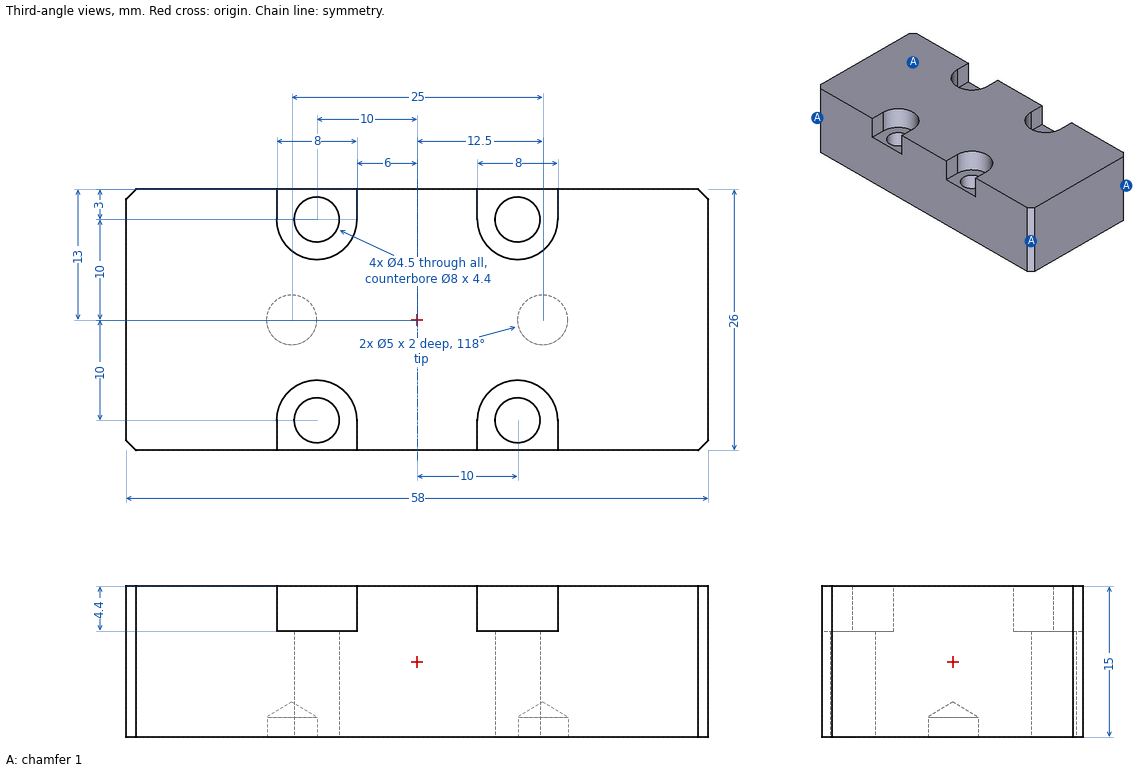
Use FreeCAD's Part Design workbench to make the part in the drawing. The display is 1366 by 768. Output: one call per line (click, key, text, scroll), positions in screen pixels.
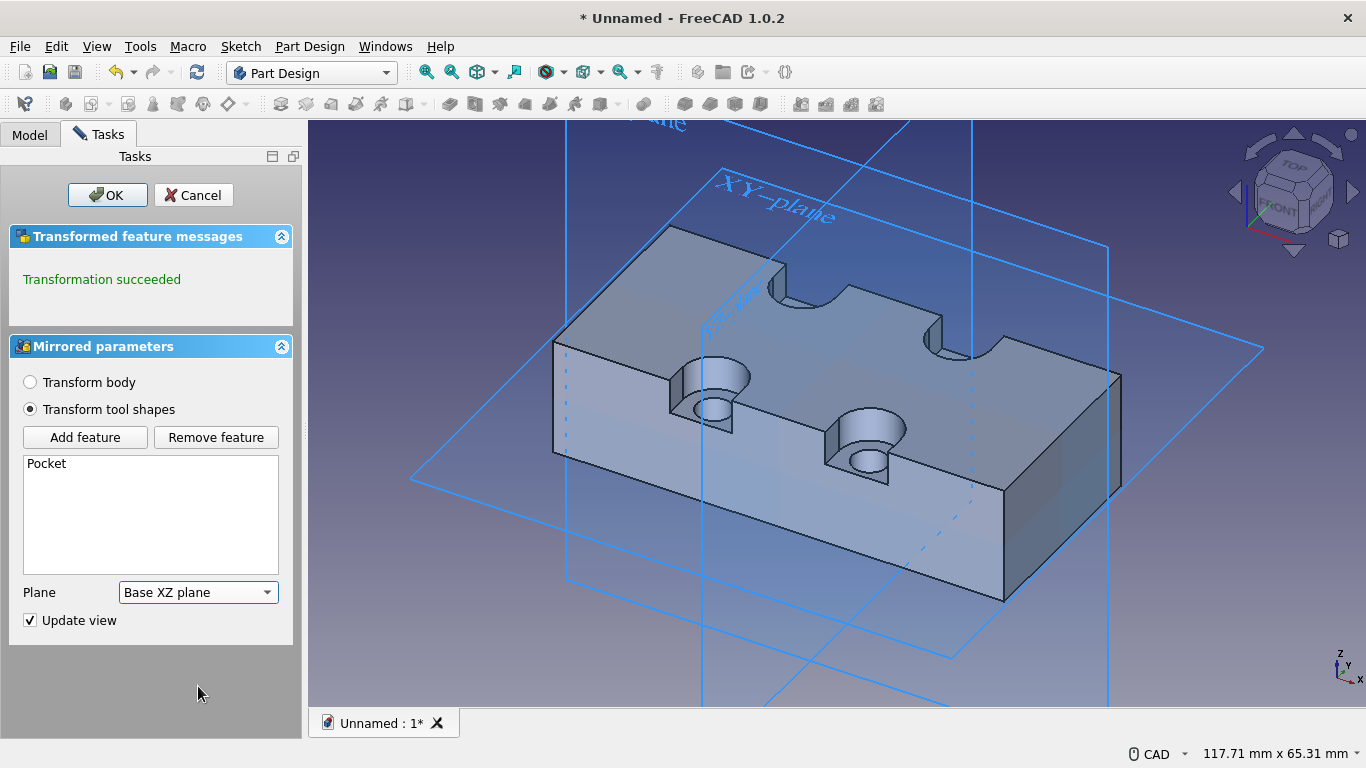
click(108, 195)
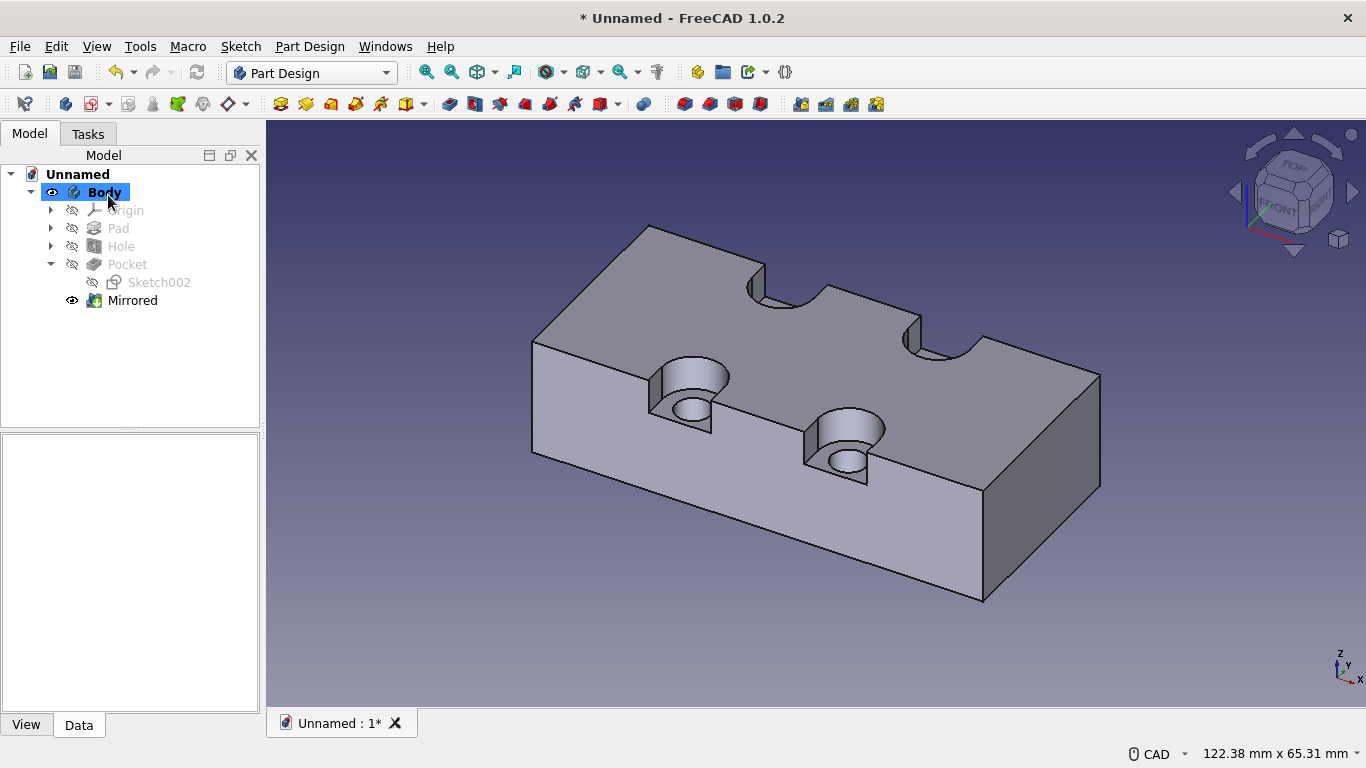
key(5)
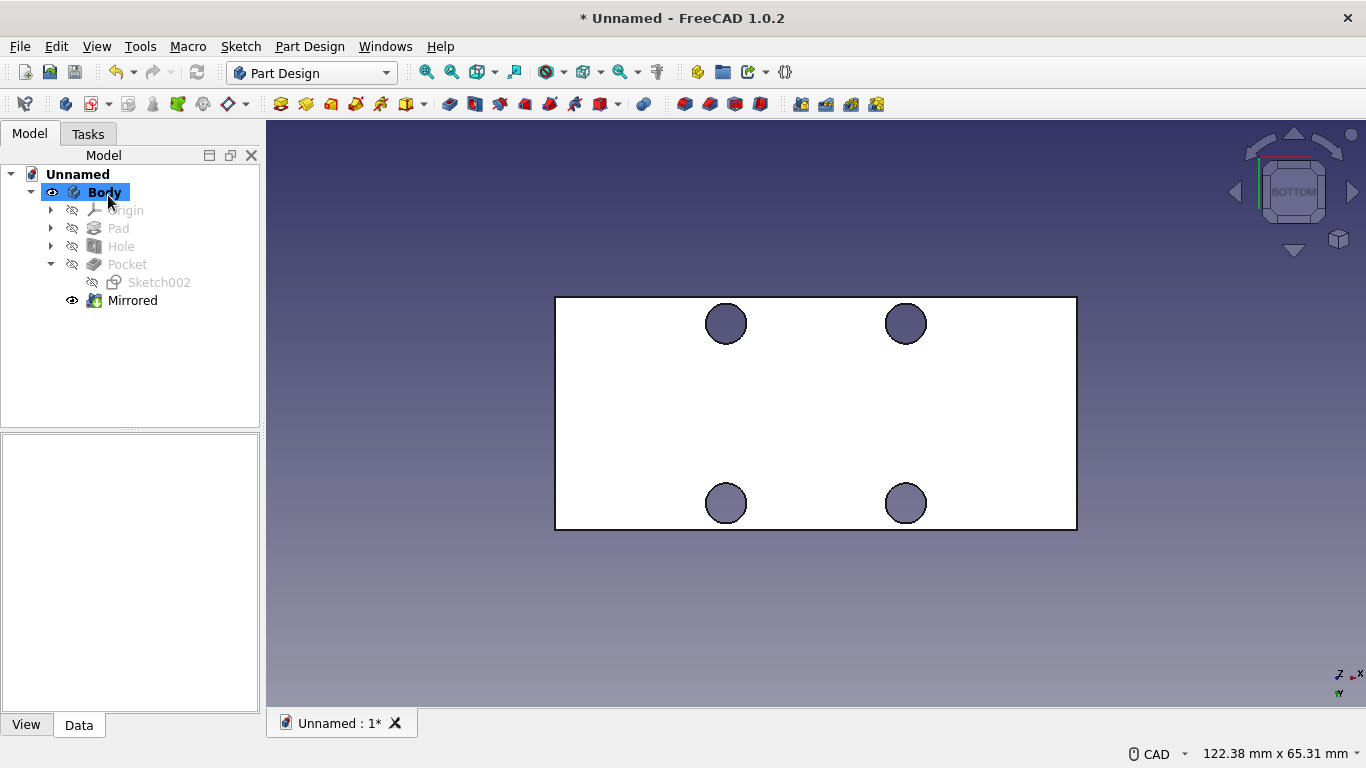
click(816, 413)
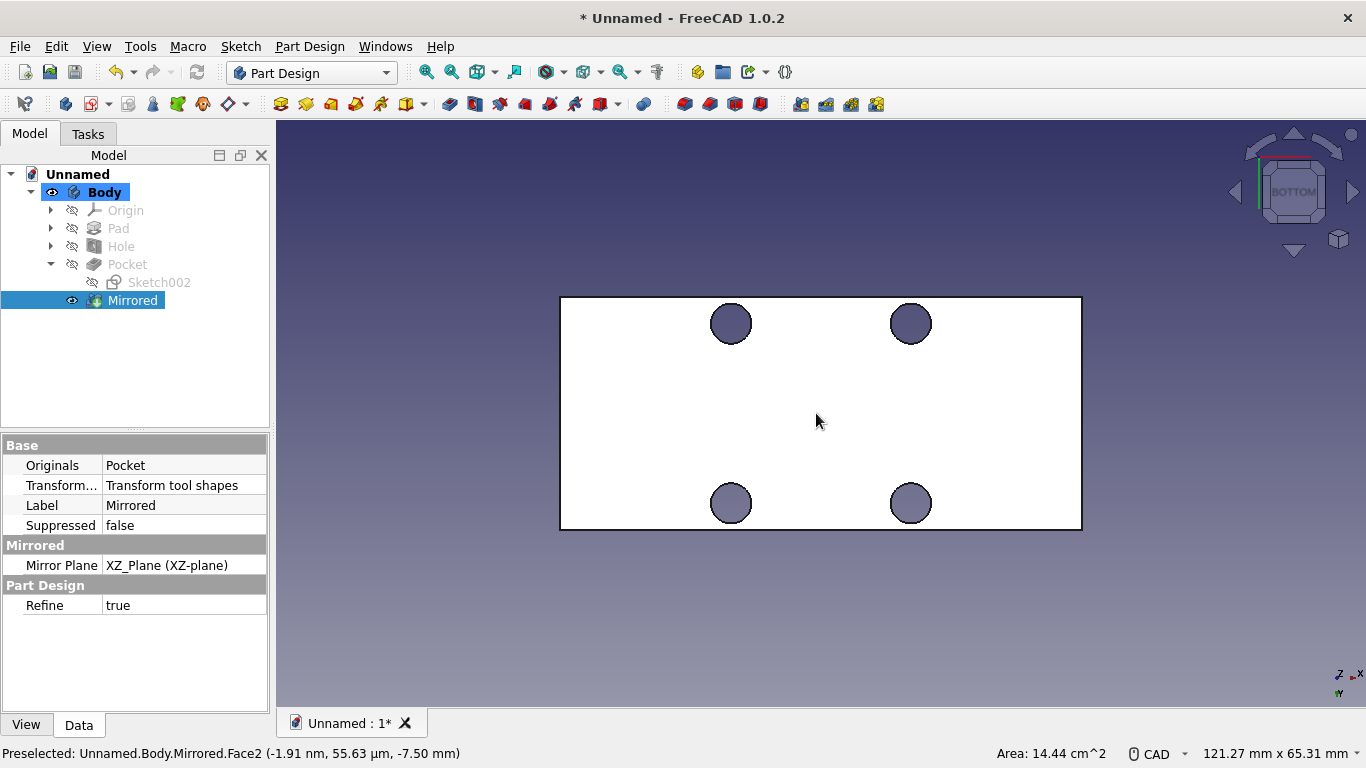
click(90, 104)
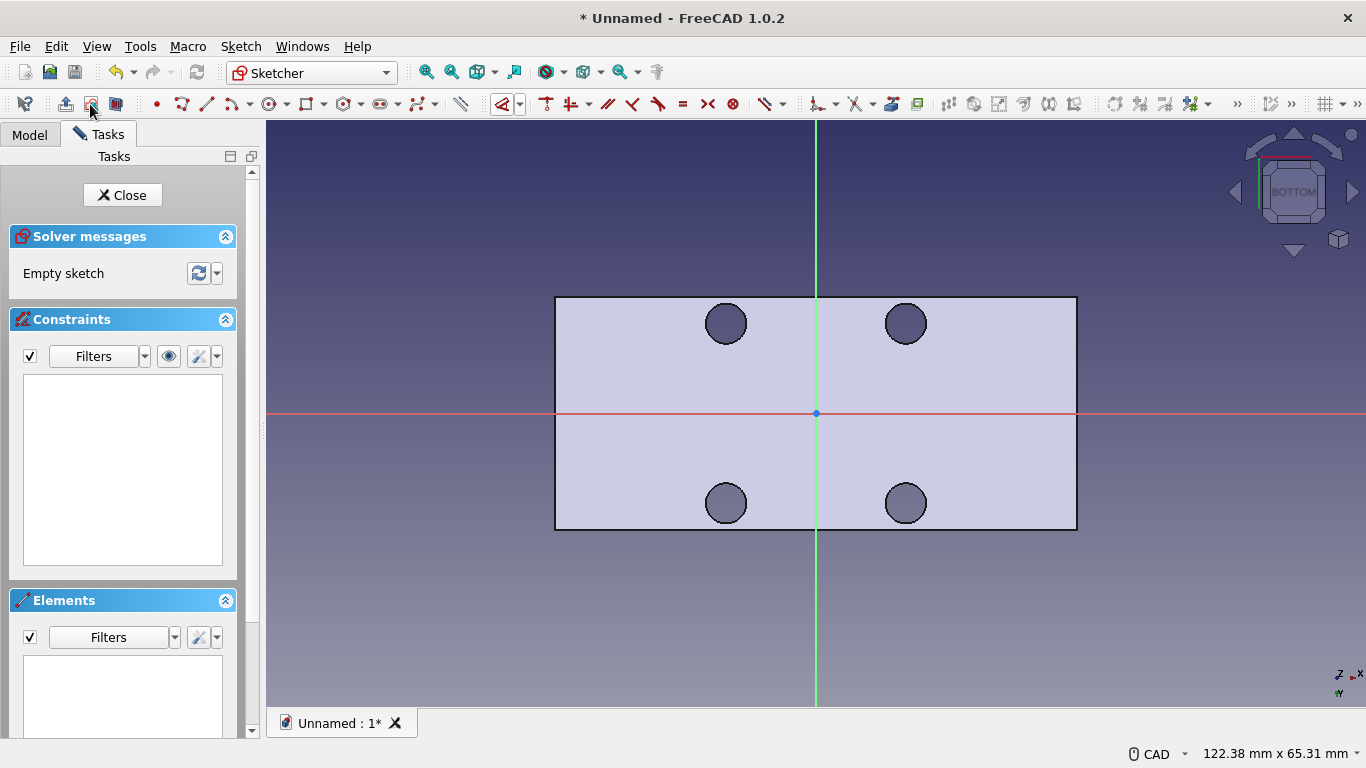
scroll(872, 414, up, 4)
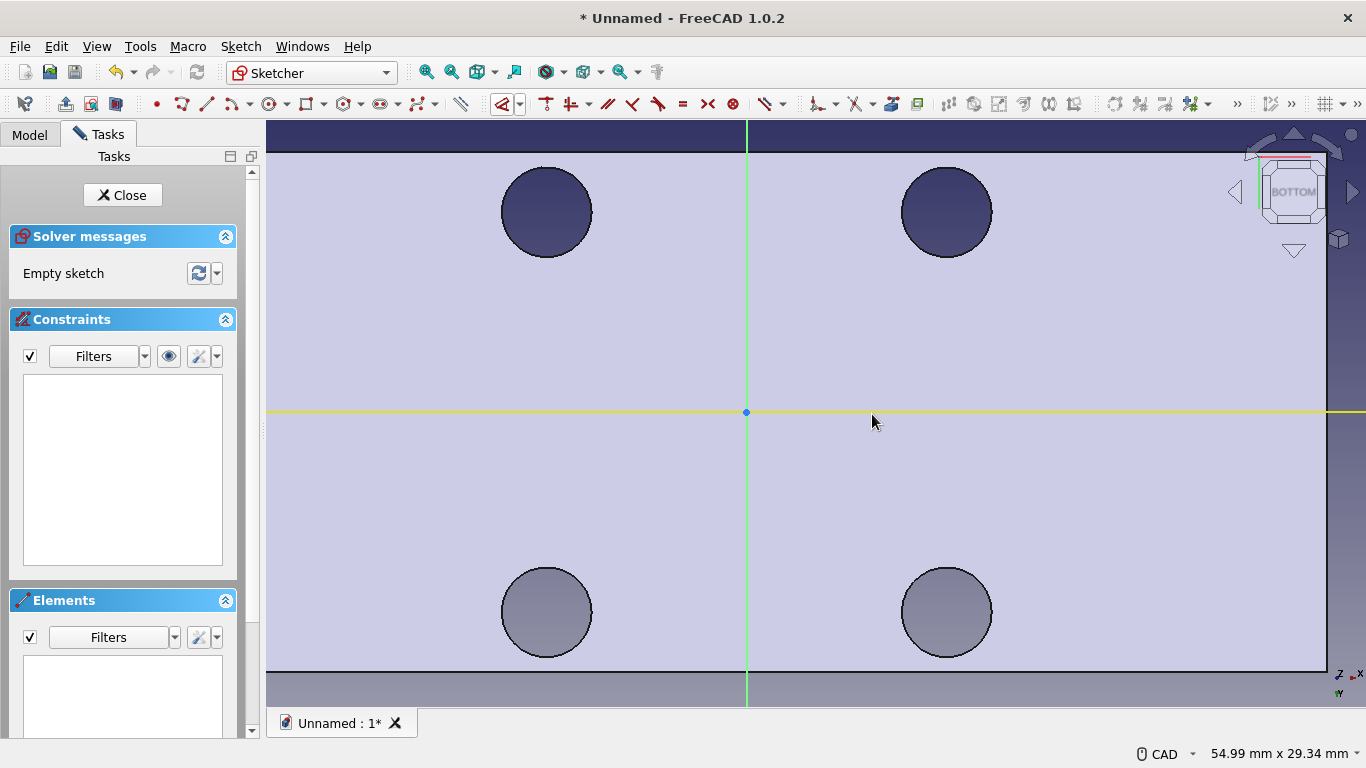
click(268, 104)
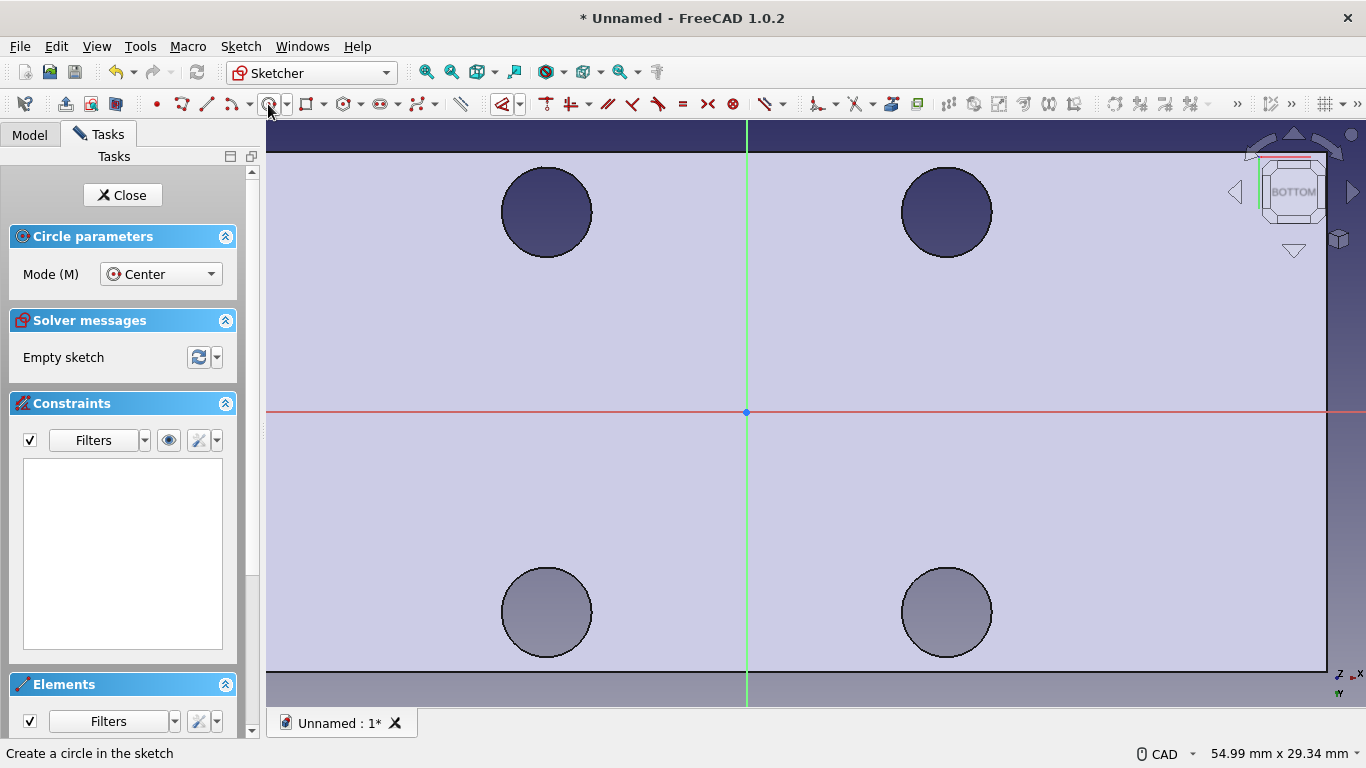
click(997, 412)
move(1032, 377)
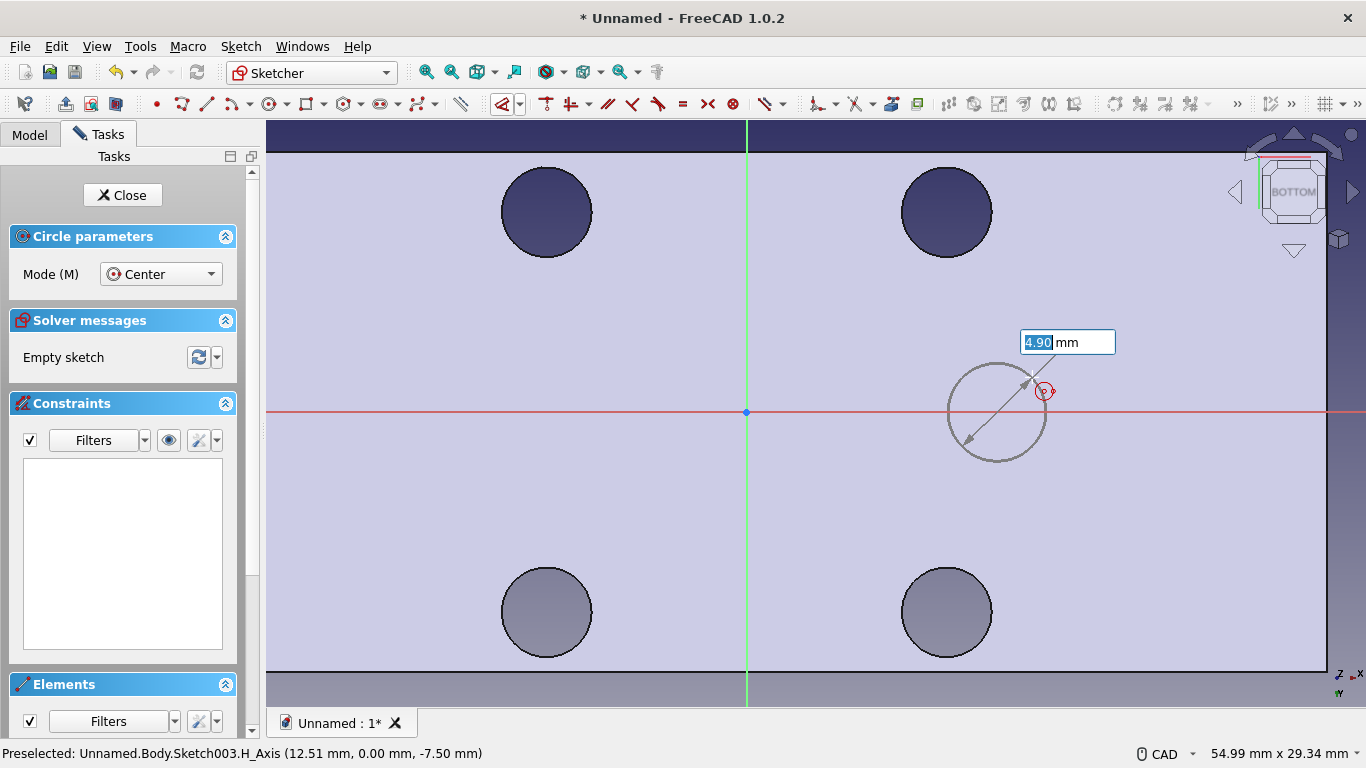
text(5)
key(Return)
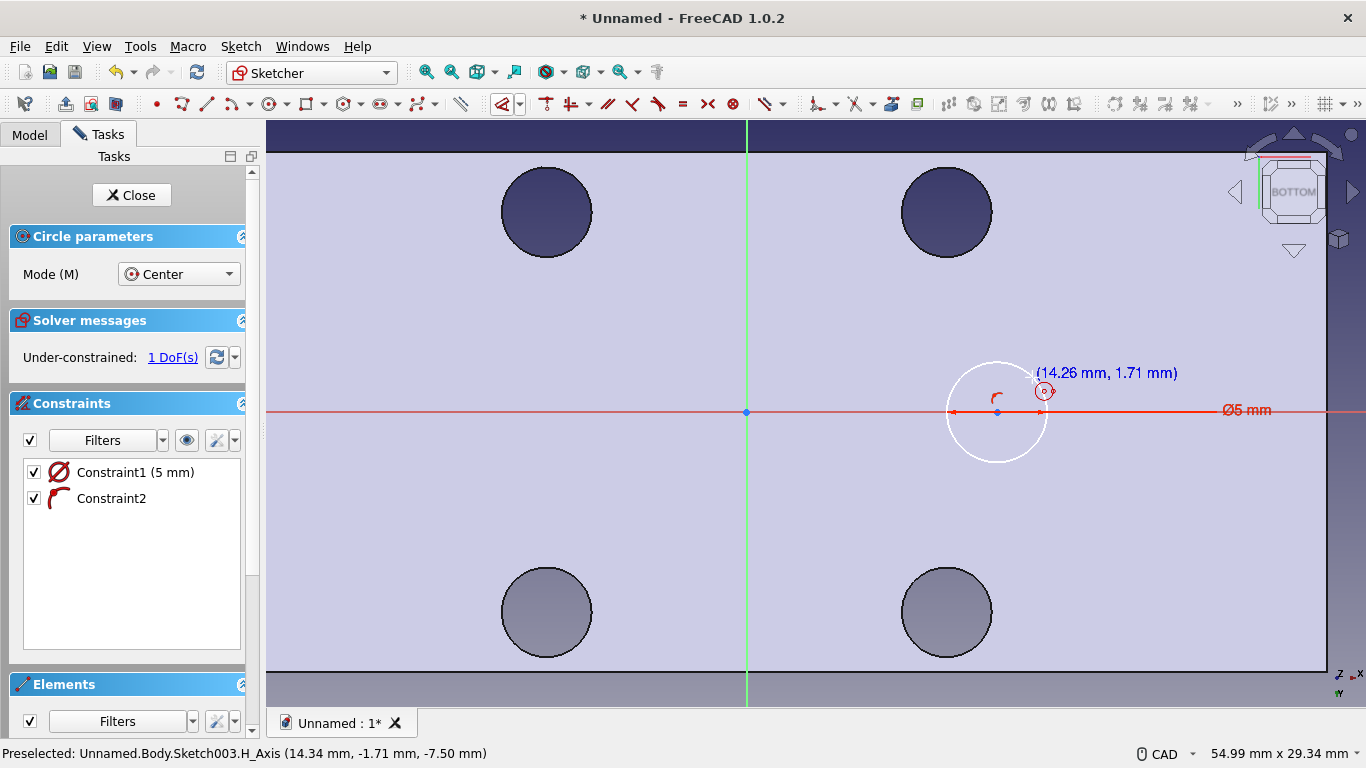
click(497, 412)
move(532, 377)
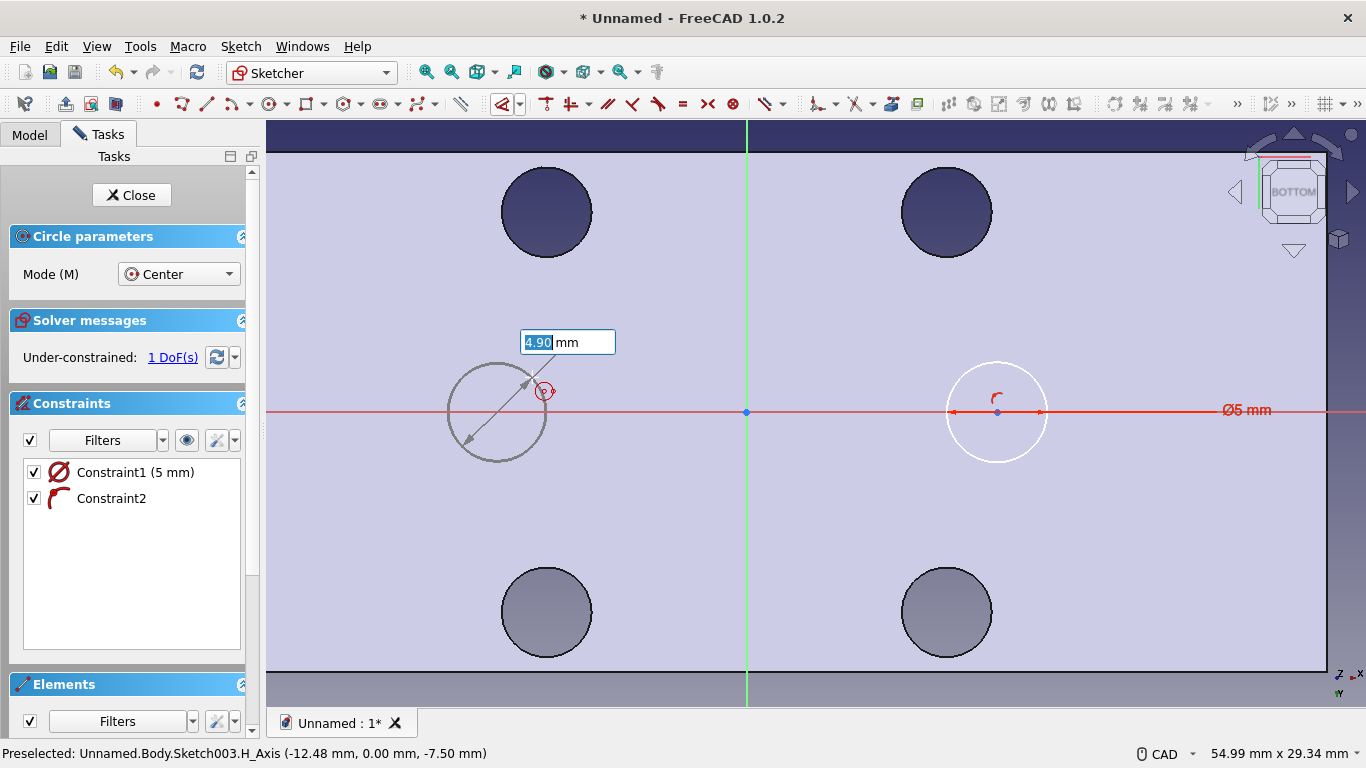
text(5)
key(Return)
key(Escape)